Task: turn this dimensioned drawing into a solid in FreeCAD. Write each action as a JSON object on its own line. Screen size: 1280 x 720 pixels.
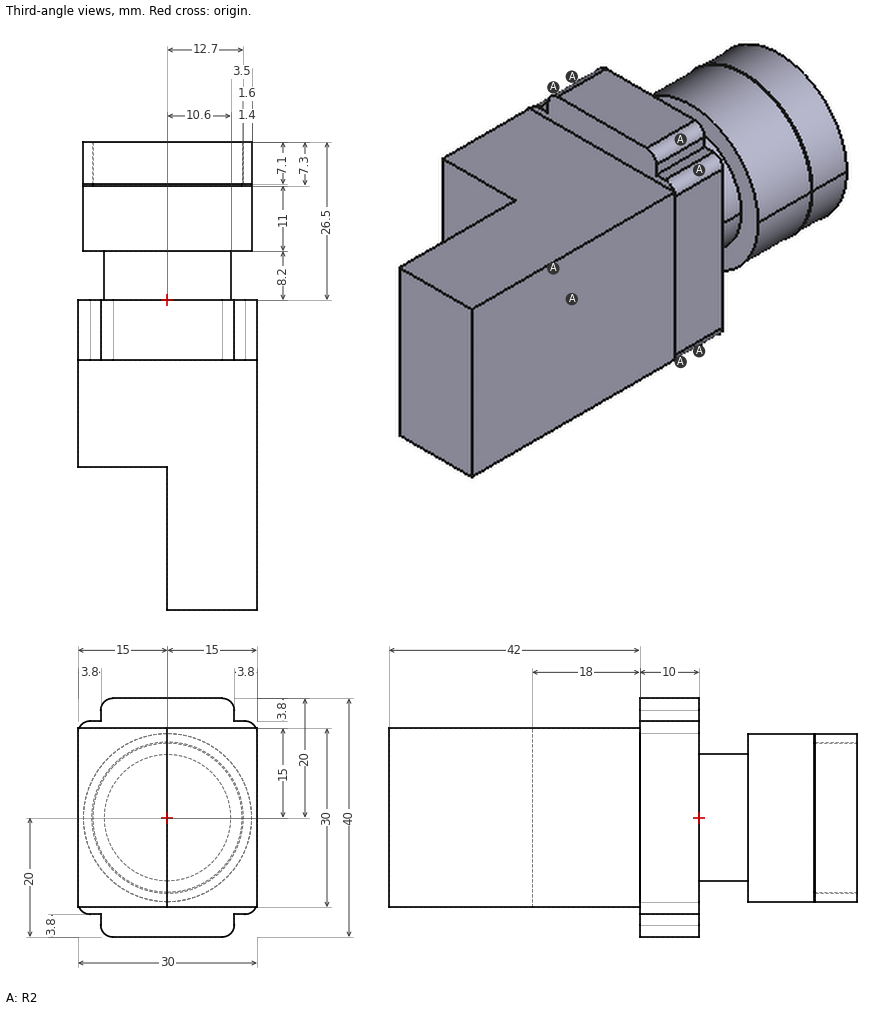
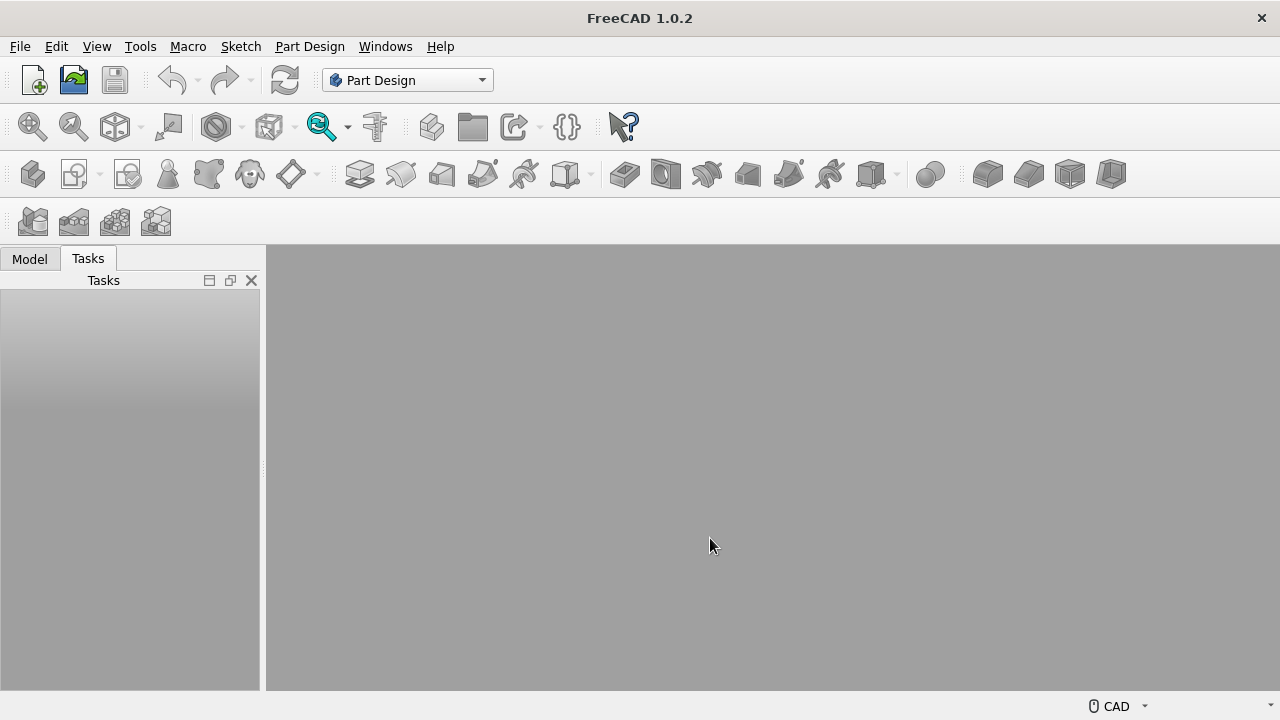
{"action": "left_click", "coordinate": [33, 80]}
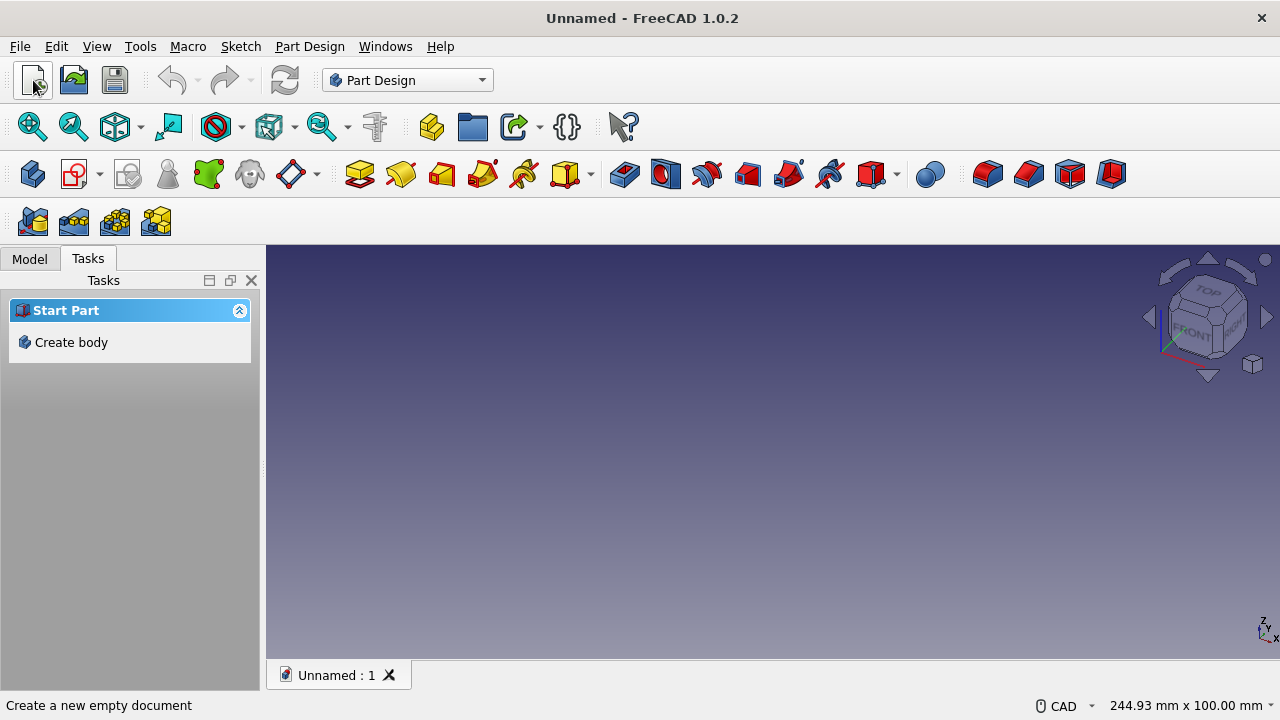
{"action": "left_click", "coordinate": [74, 174]}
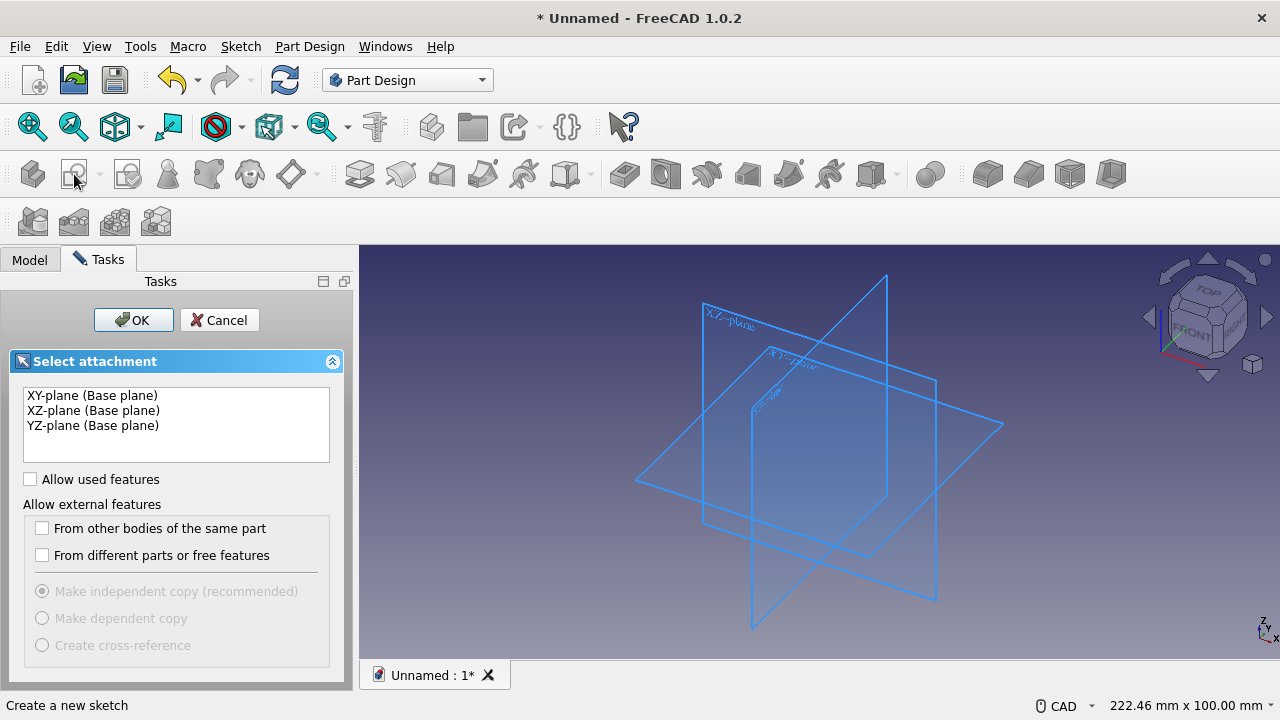
{"action": "left_click", "coordinate": [84, 396]}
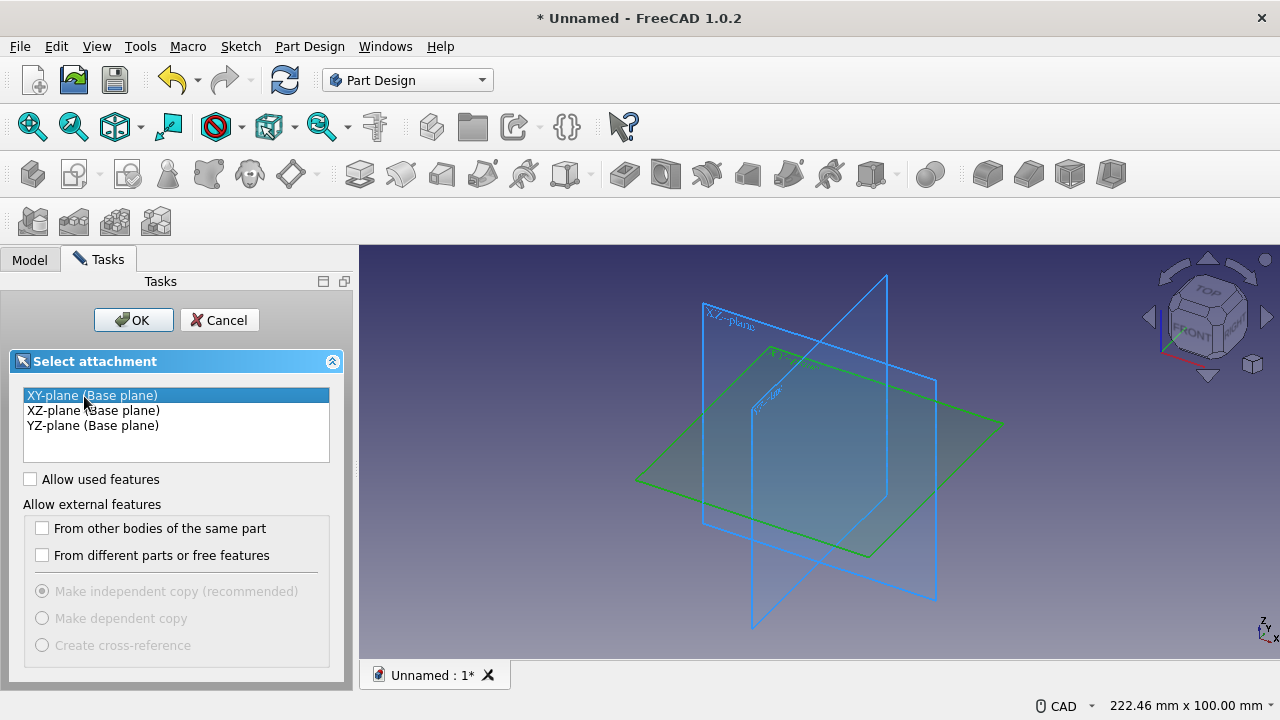
{"action": "left_click", "coordinate": [134, 320]}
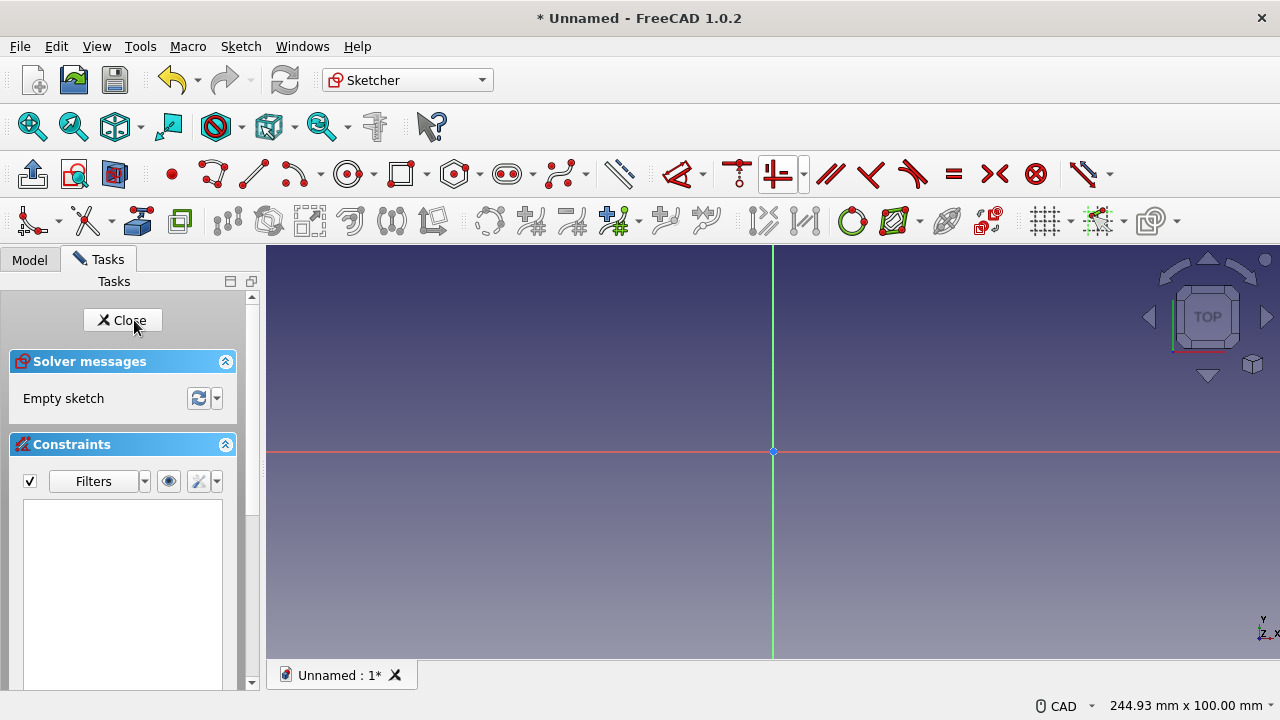
{"action": "scroll", "coordinate": [882, 352], "scroll_direction": "up", "scroll_amount": 4}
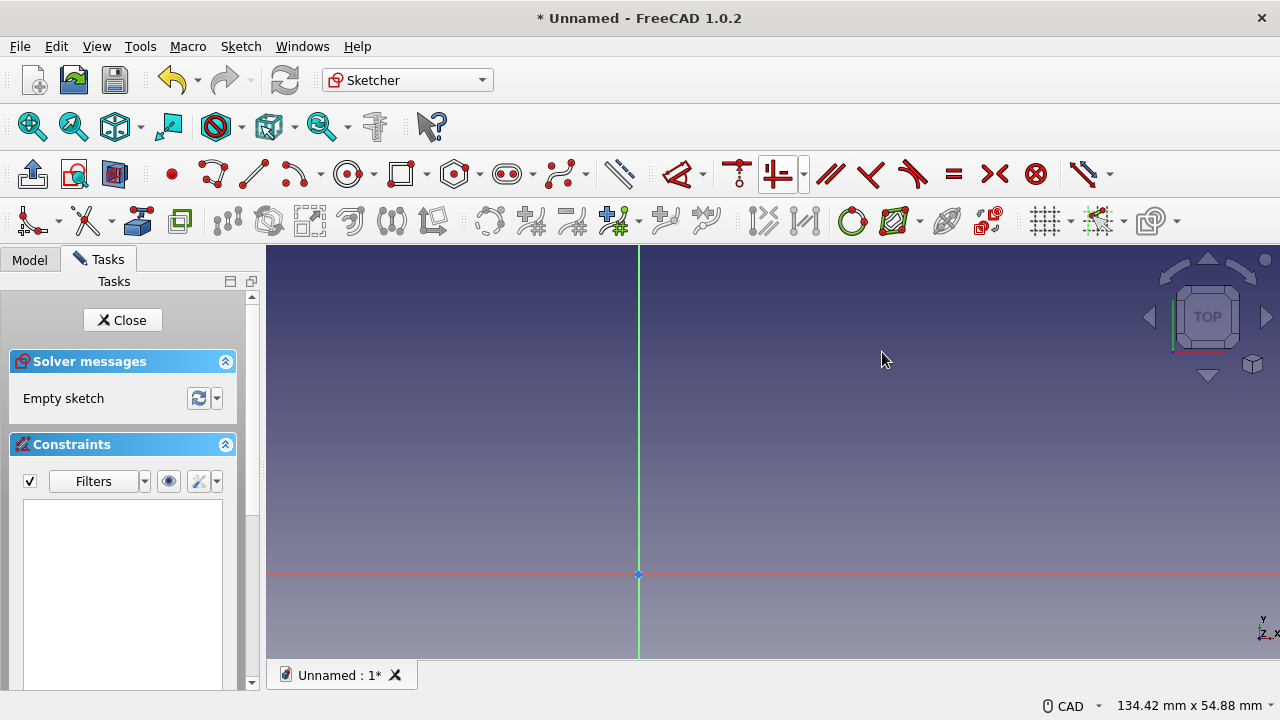
{"action": "left_click", "coordinate": [213, 174]}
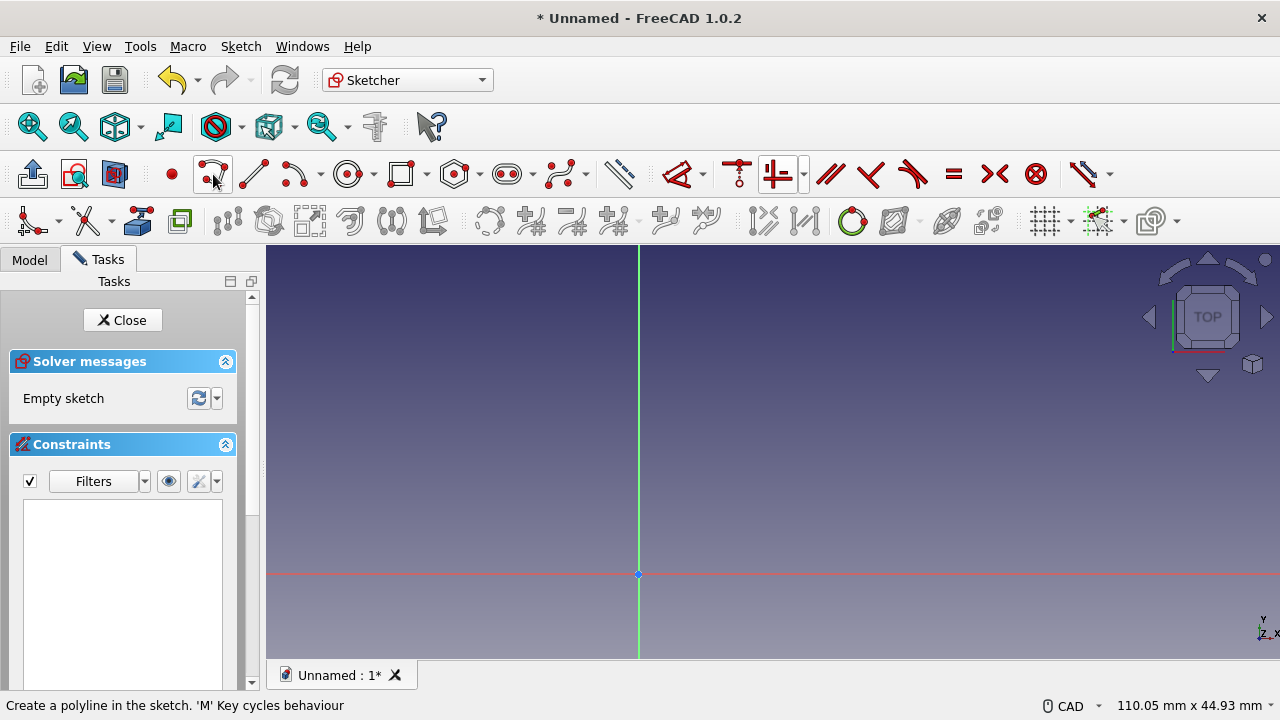
{"action": "left_click", "coordinate": [639, 574]}
{"action": "left_click", "coordinate": [736, 565]}
{"action": "left_click", "coordinate": [736, 499]}
{"action": "left_click", "coordinate": [769, 499]}
{"action": "left_click", "coordinate": [769, 397]}
{"action": "left_click", "coordinate": [754, 397]}
{"action": "left_click", "coordinate": [754, 330]}
{"action": "left_click", "coordinate": [648, 330]}
{"action": "left_click", "coordinate": [639, 574]}
{"action": "key", "text": "Escape"}
{"action": "key", "text": "Escape"}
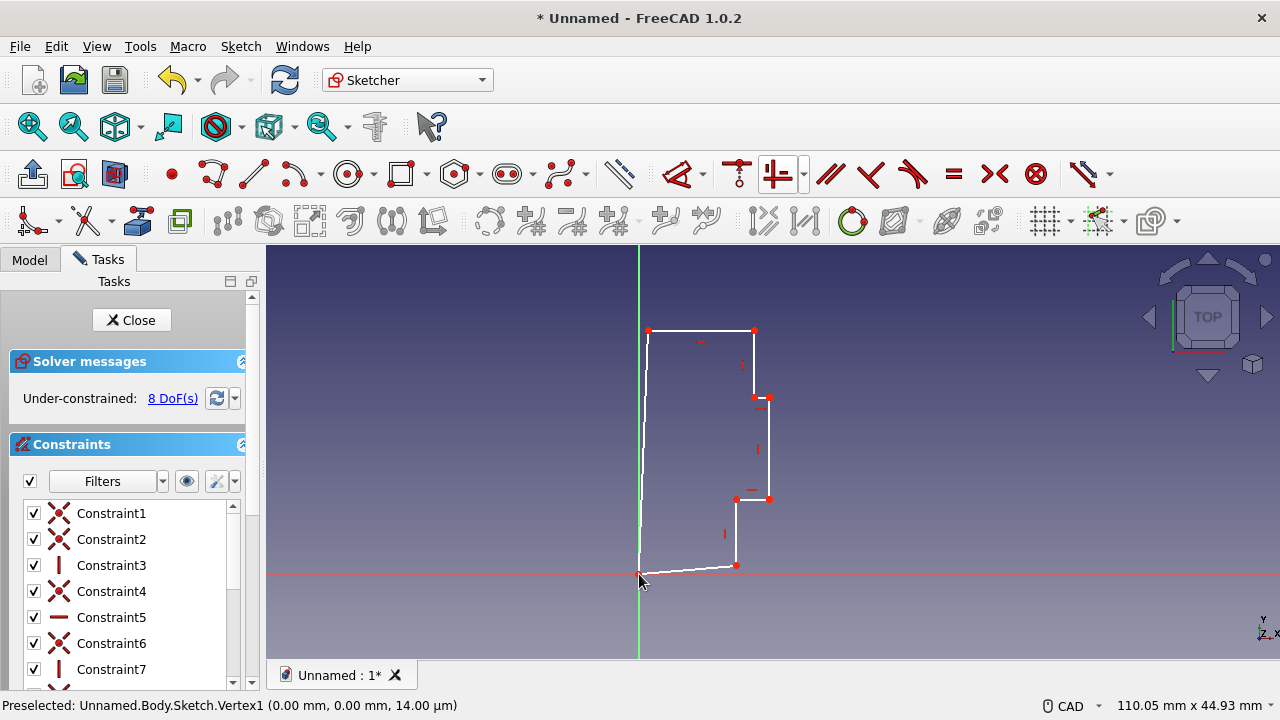
{"action": "left_click", "coordinate": [668, 572]}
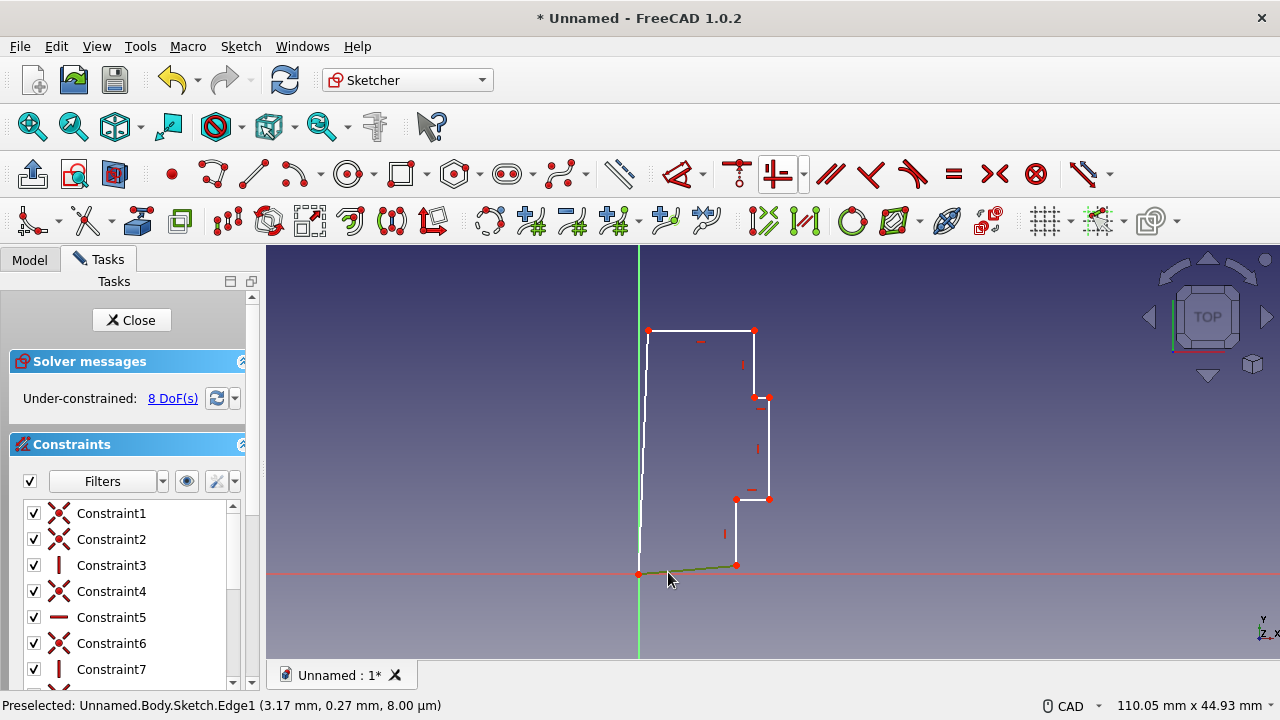
{"action": "key", "text": "h"}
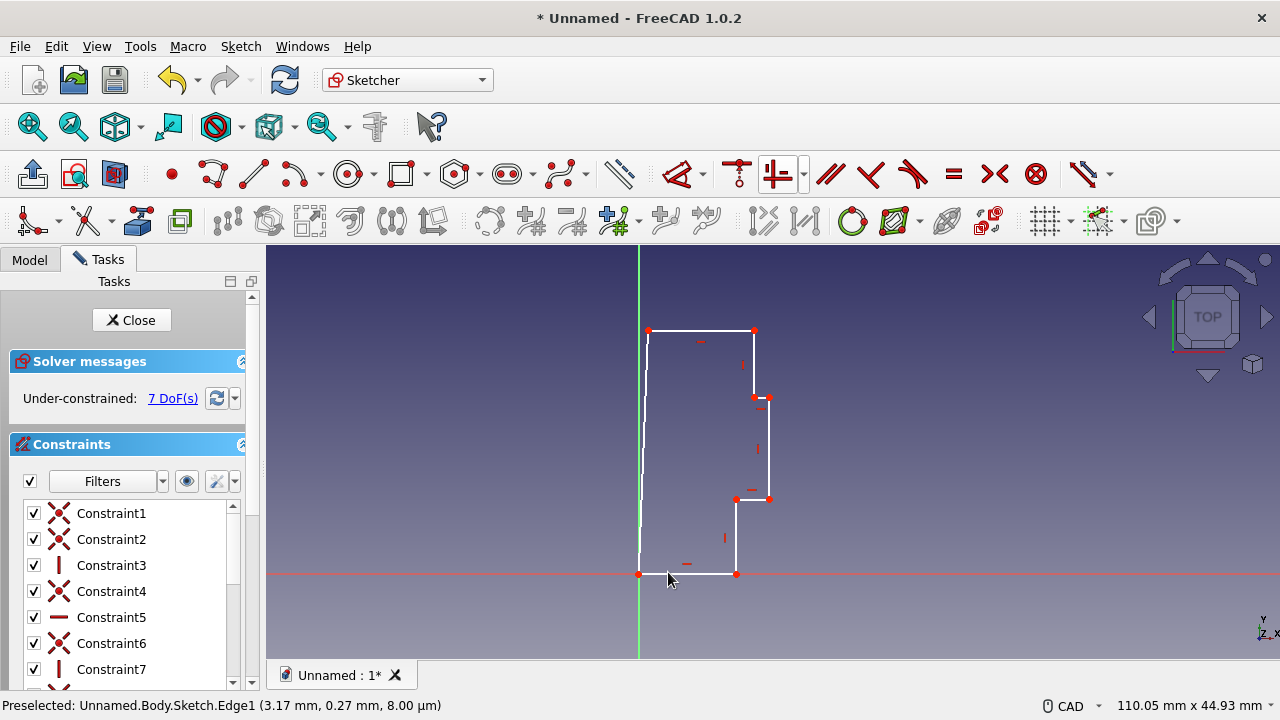
{"action": "left_click", "coordinate": [641, 501]}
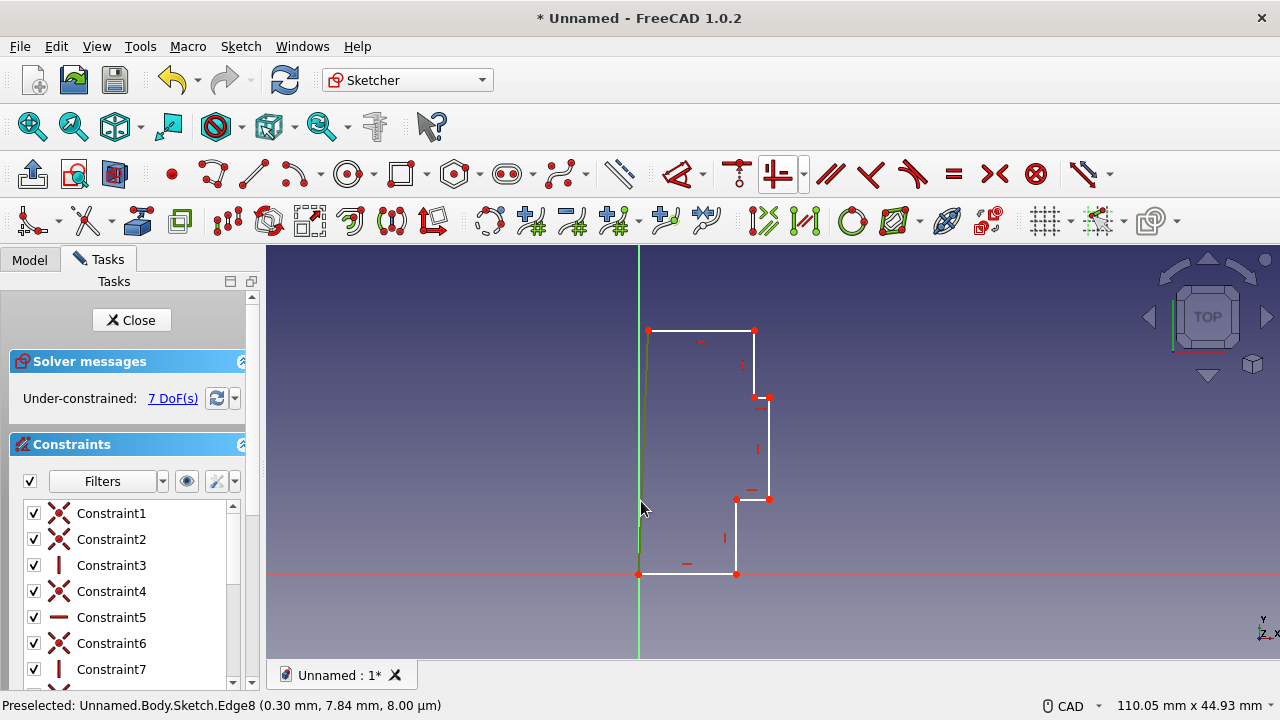
{"action": "key", "text": "v"}